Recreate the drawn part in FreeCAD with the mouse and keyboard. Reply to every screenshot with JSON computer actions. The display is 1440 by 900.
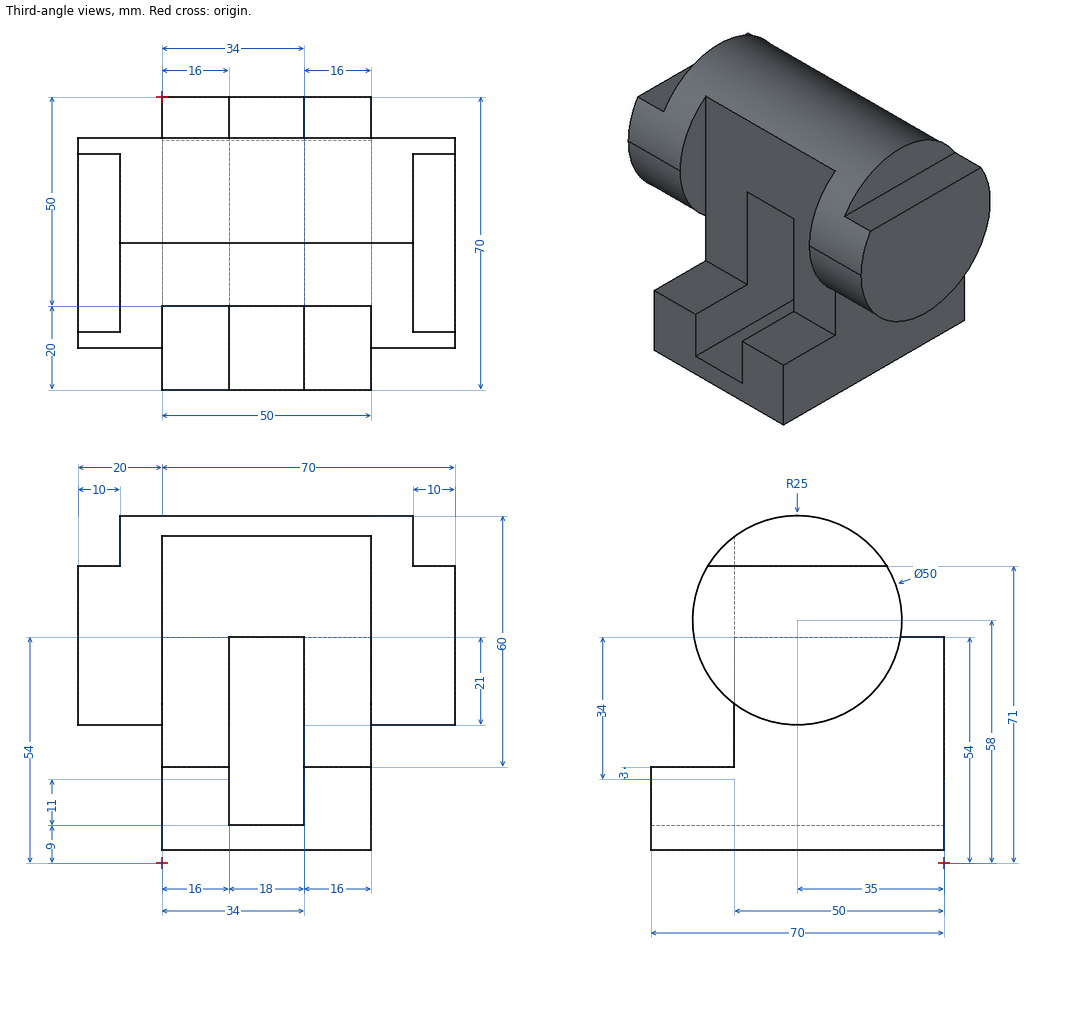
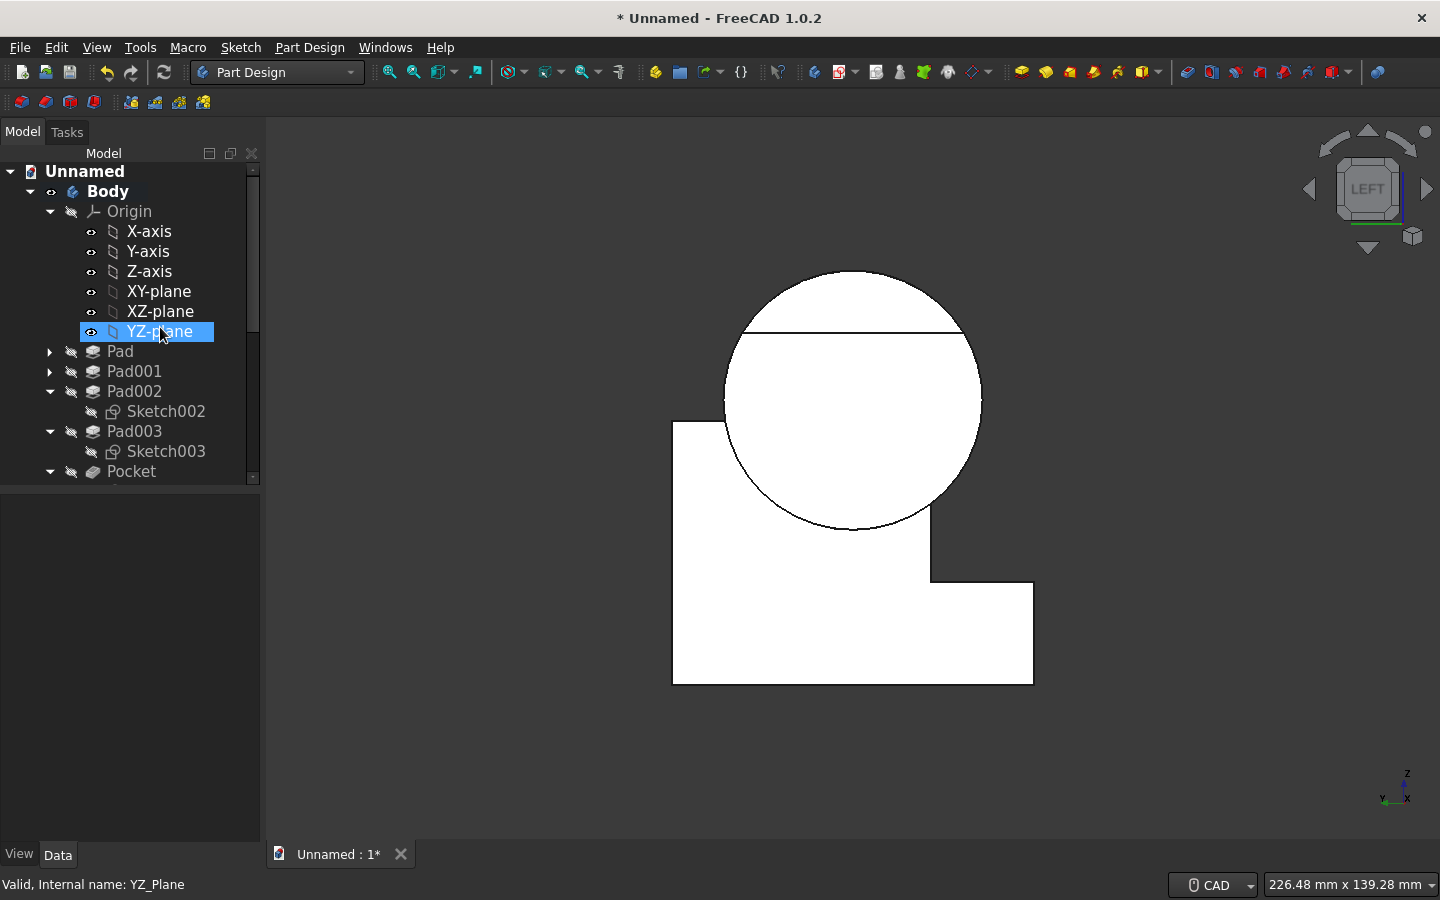
{"action": "left_click", "coordinate": [136, 332]}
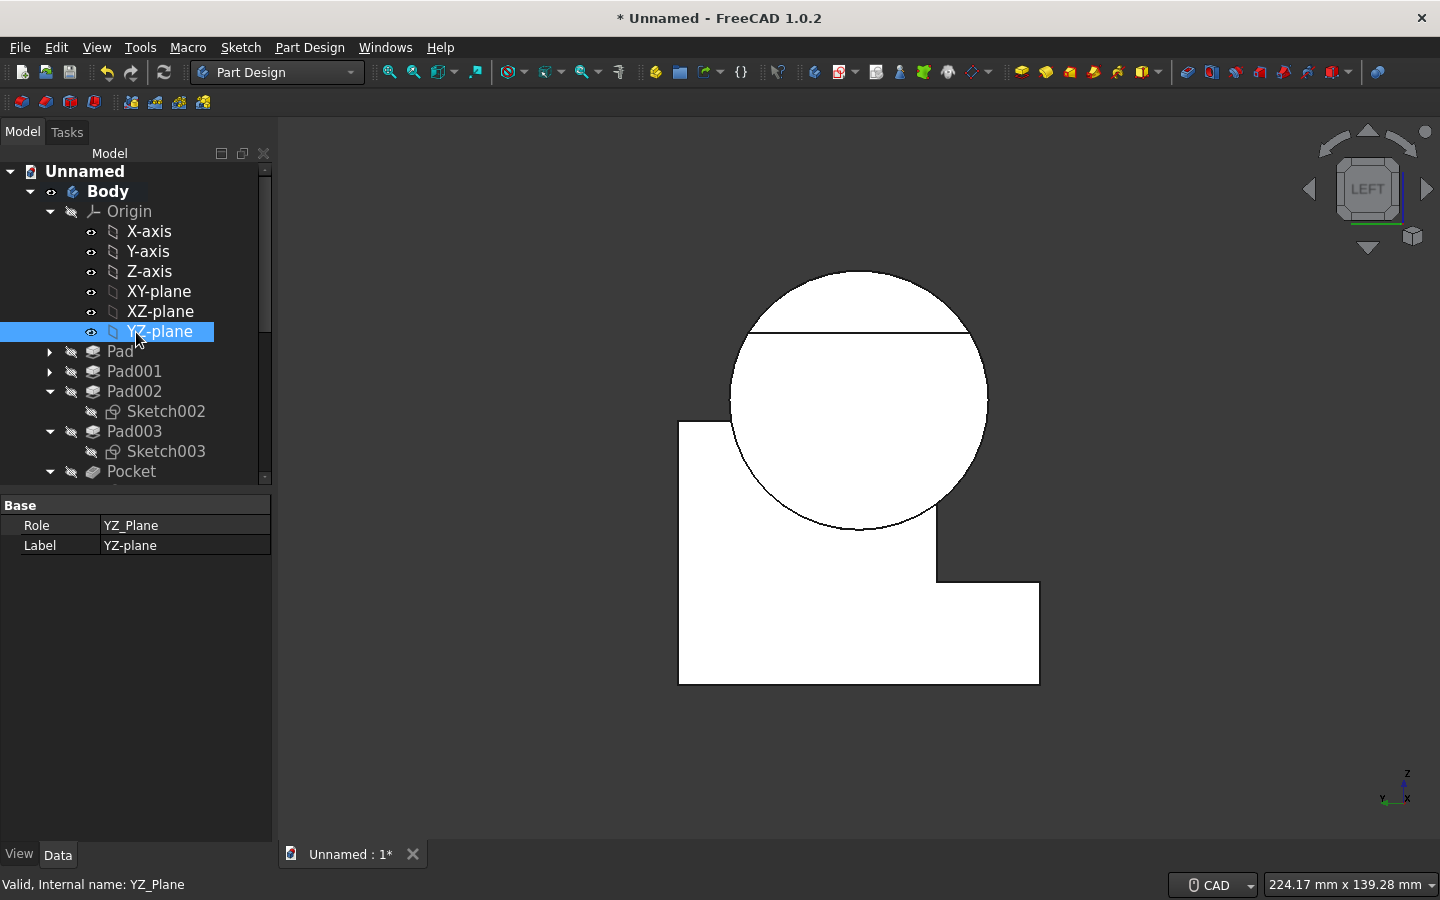
{"action": "left_click", "coordinate": [972, 72]}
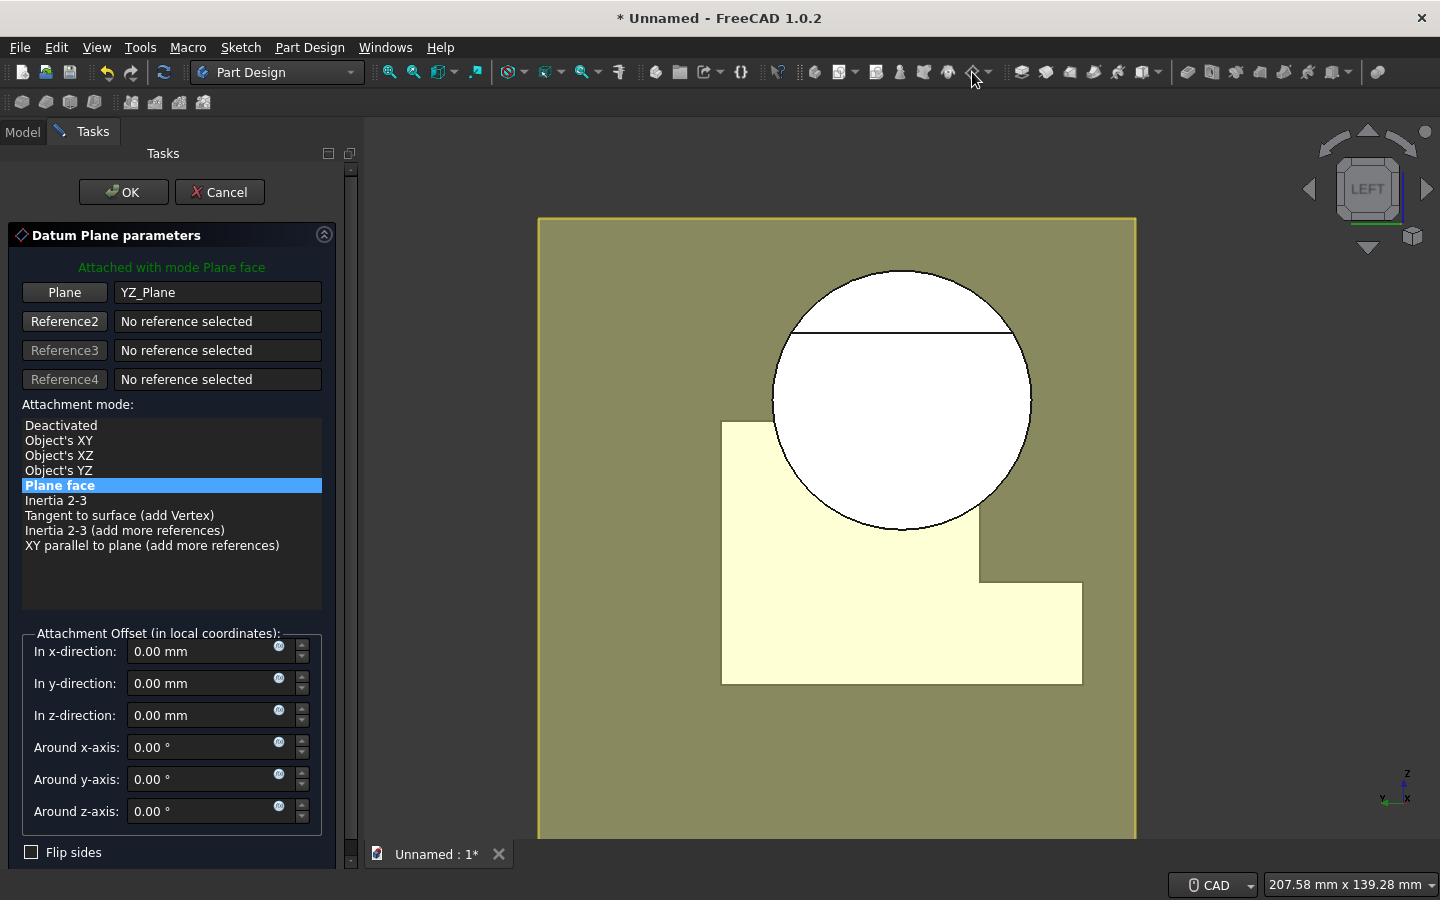
{"action": "triple_click", "coordinate": [210, 715]}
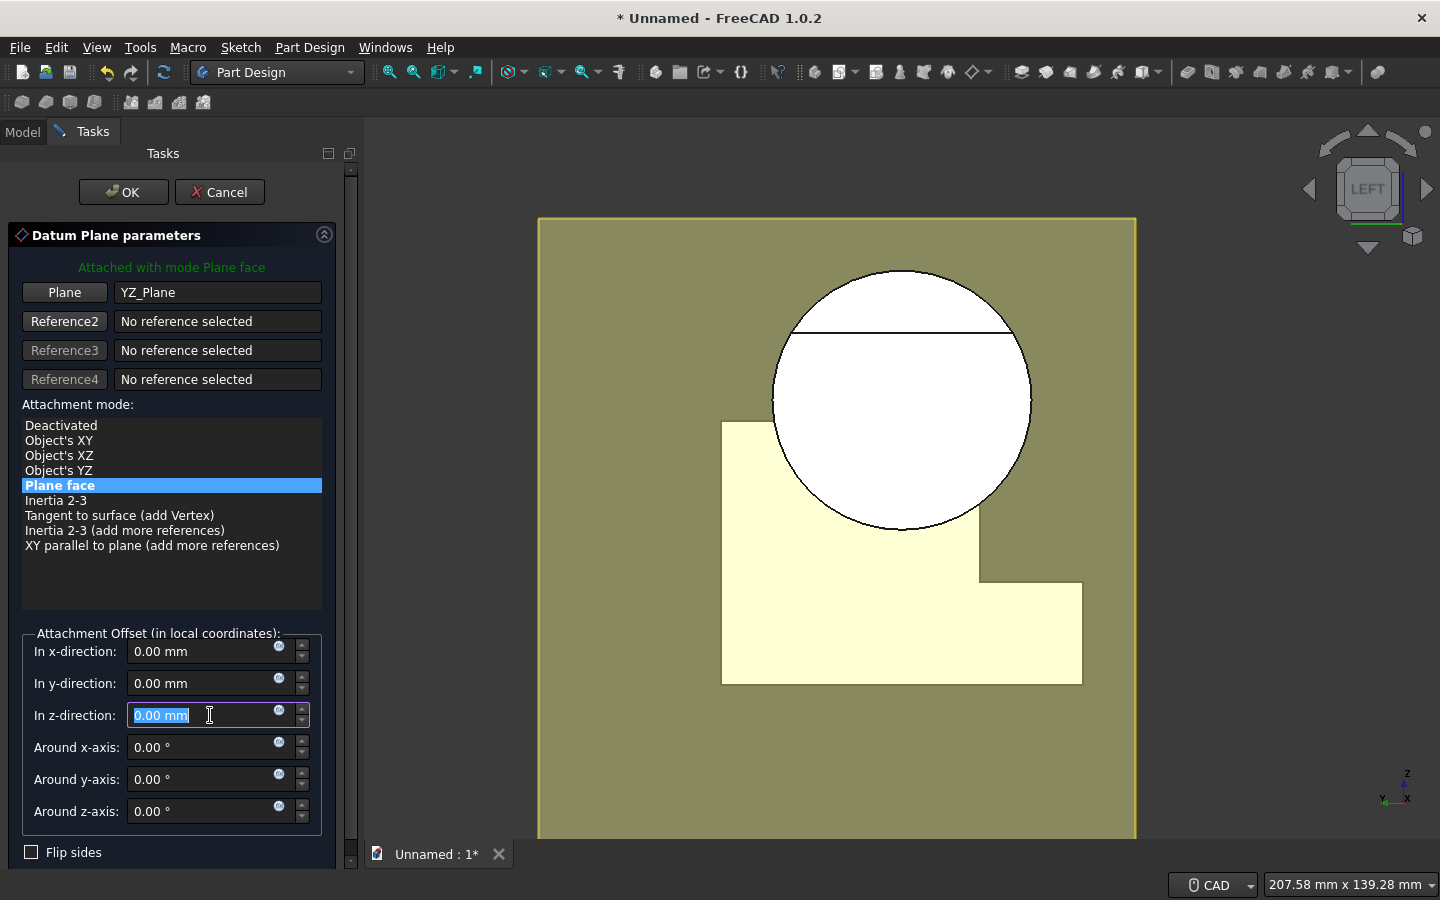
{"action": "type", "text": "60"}
{"action": "key", "text": "Tab"}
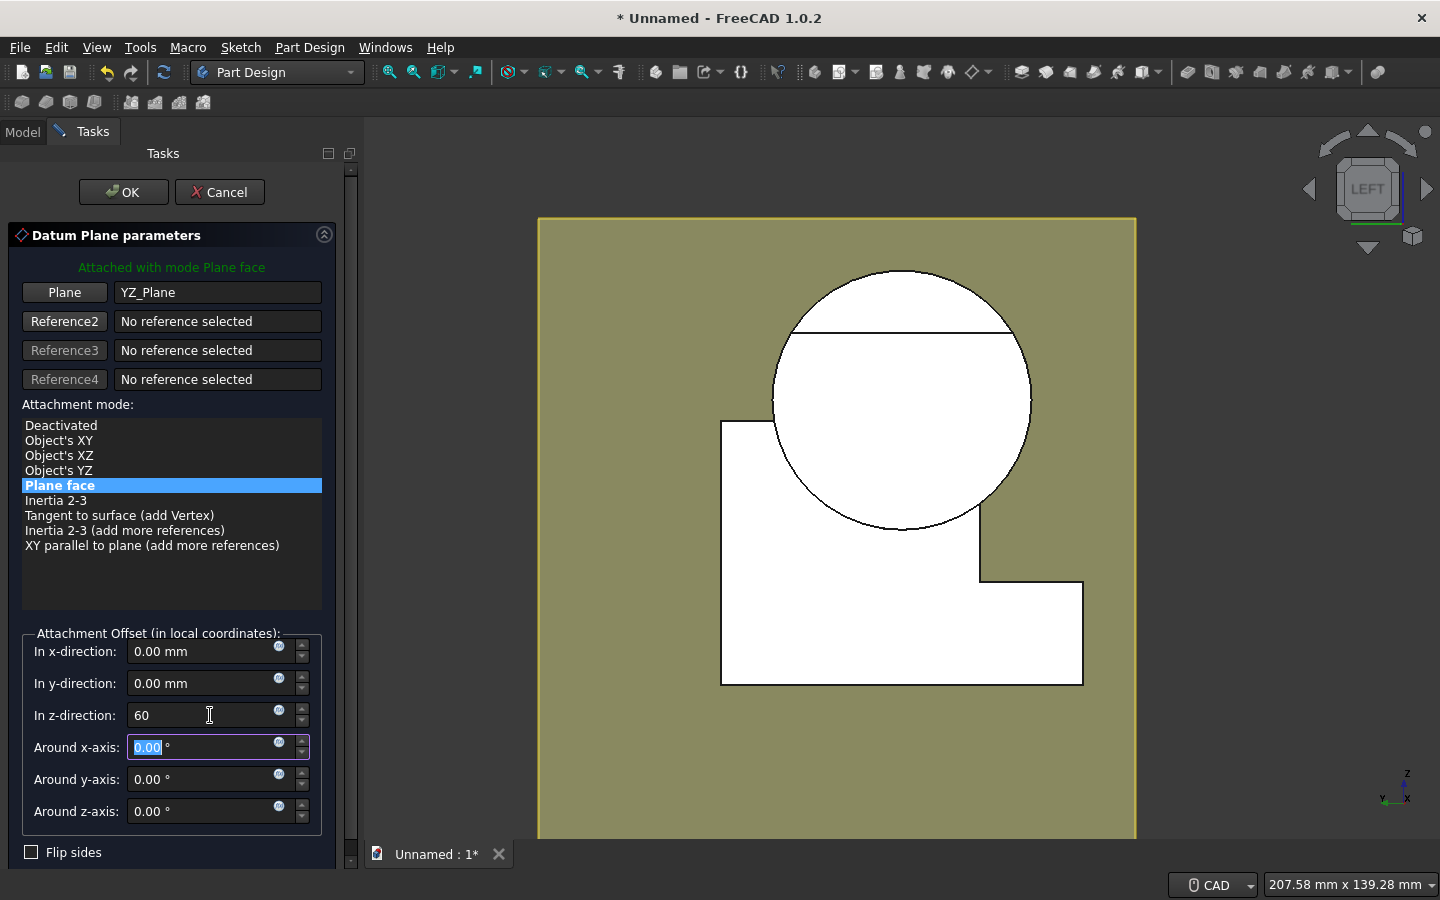
{"action": "left_click", "coordinate": [124, 192]}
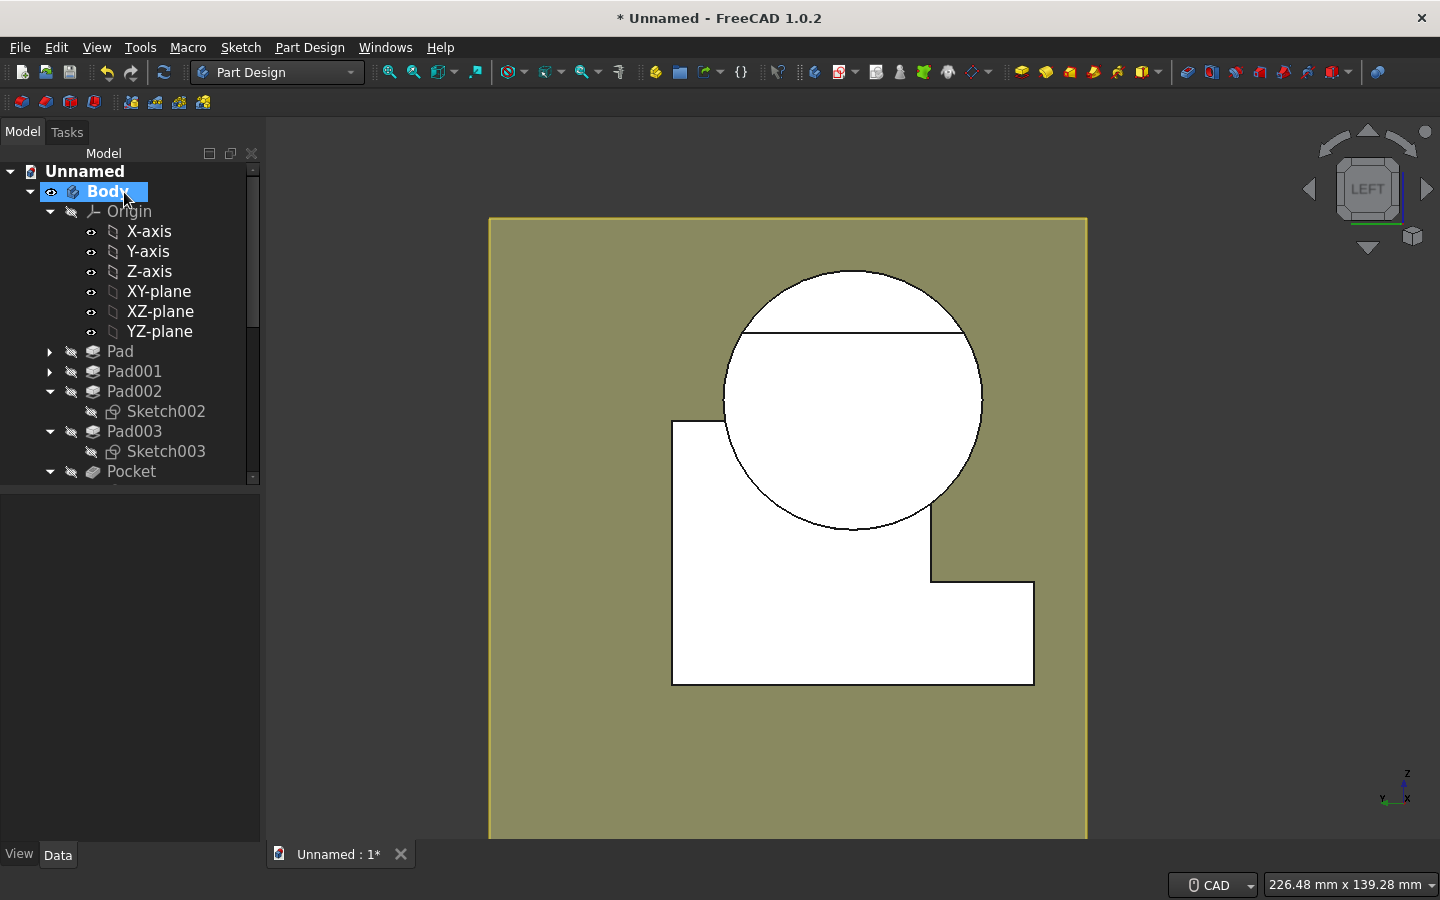
{"action": "scroll", "coordinate": [100, 327], "scroll_direction": "down", "scroll_amount": 3}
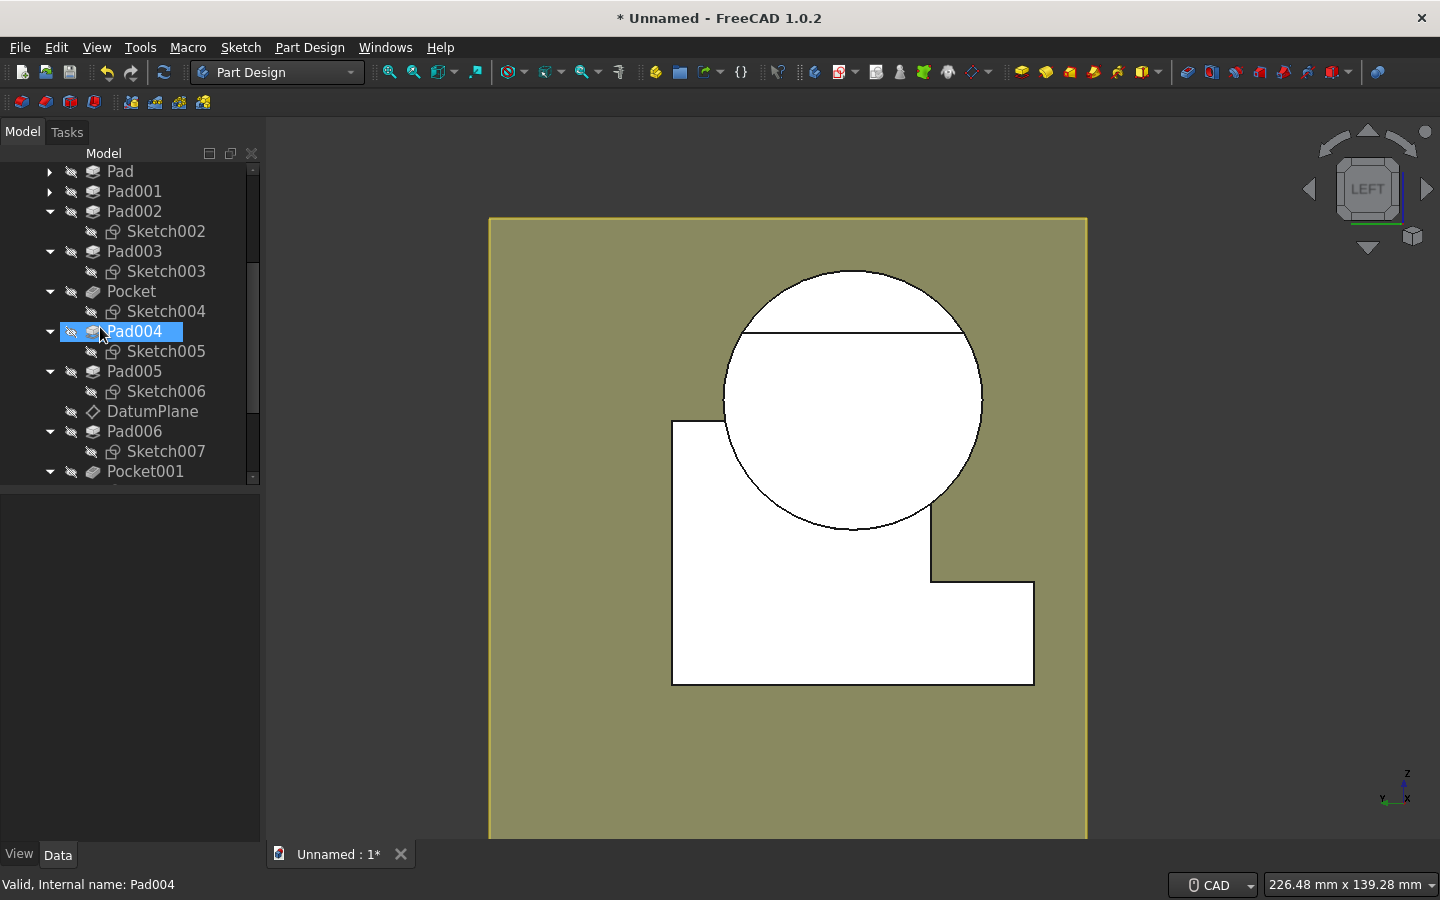
{"action": "scroll", "coordinate": [140, 327], "scroll_direction": "up", "scroll_amount": 15}